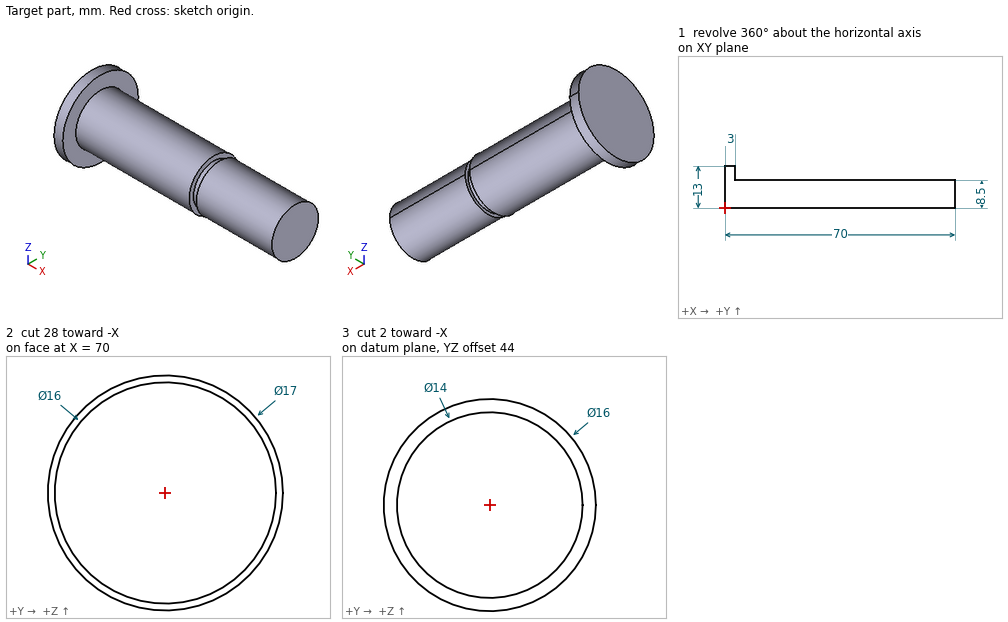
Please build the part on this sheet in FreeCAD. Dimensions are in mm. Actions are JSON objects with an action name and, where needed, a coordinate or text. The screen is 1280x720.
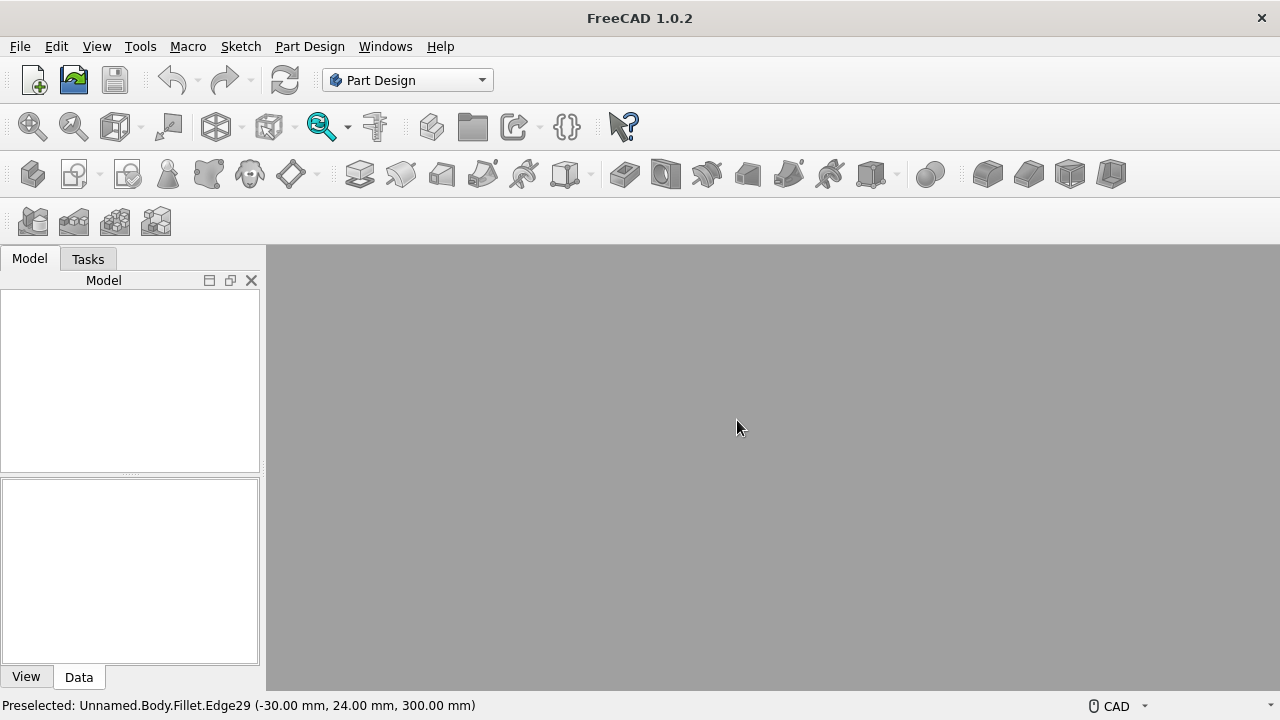
{"action": "key", "text": "ctrl+n"}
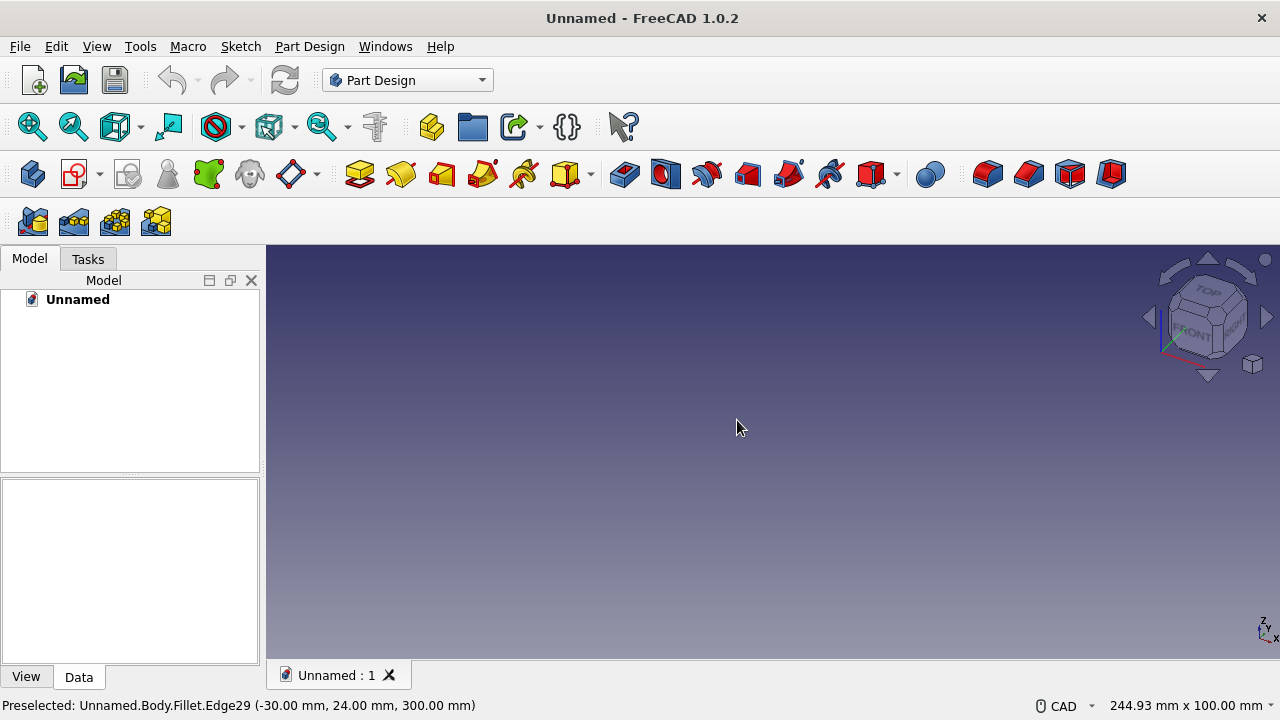
{"action": "left_click", "coordinate": [74, 174]}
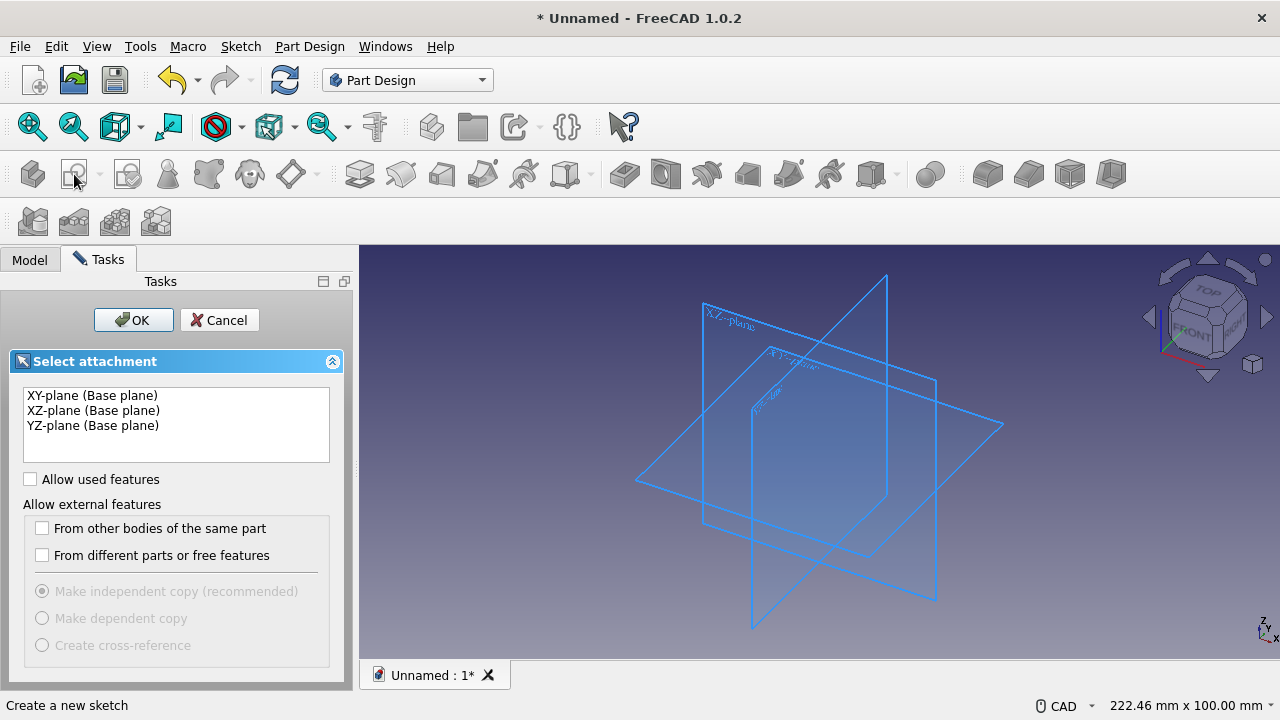
{"action": "left_click", "coordinate": [84, 396]}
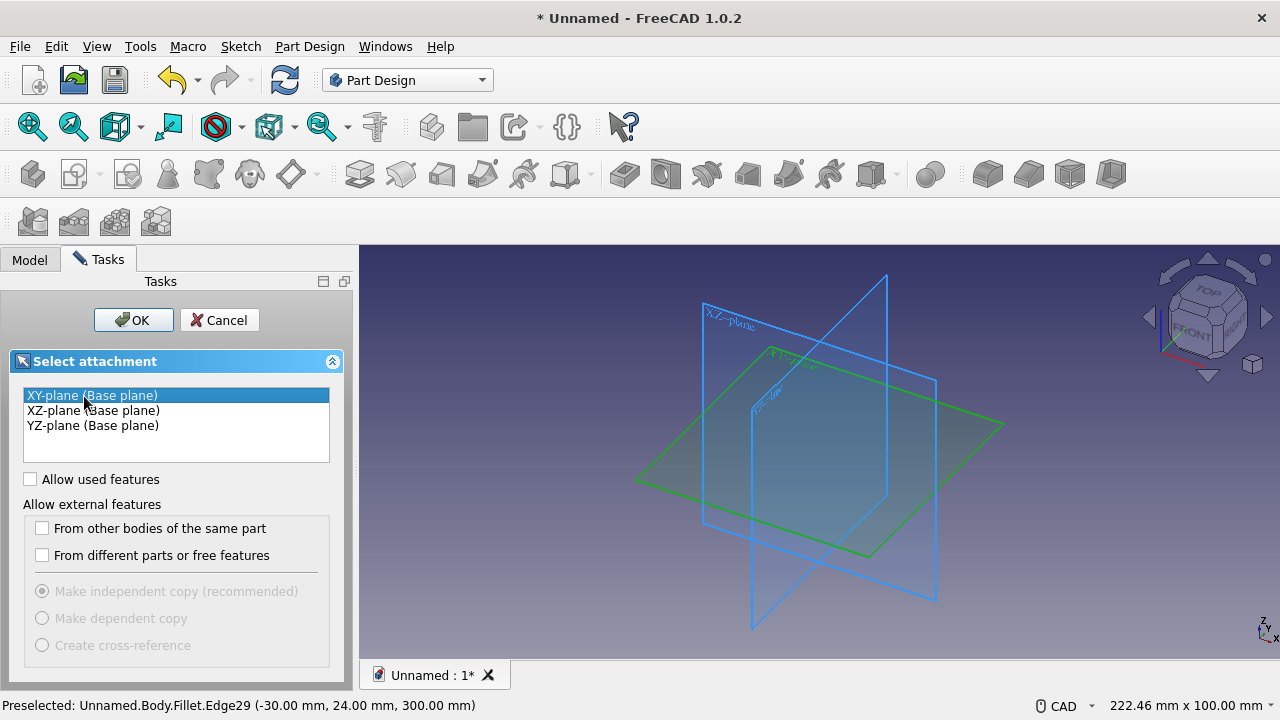
{"action": "left_click", "coordinate": [134, 320]}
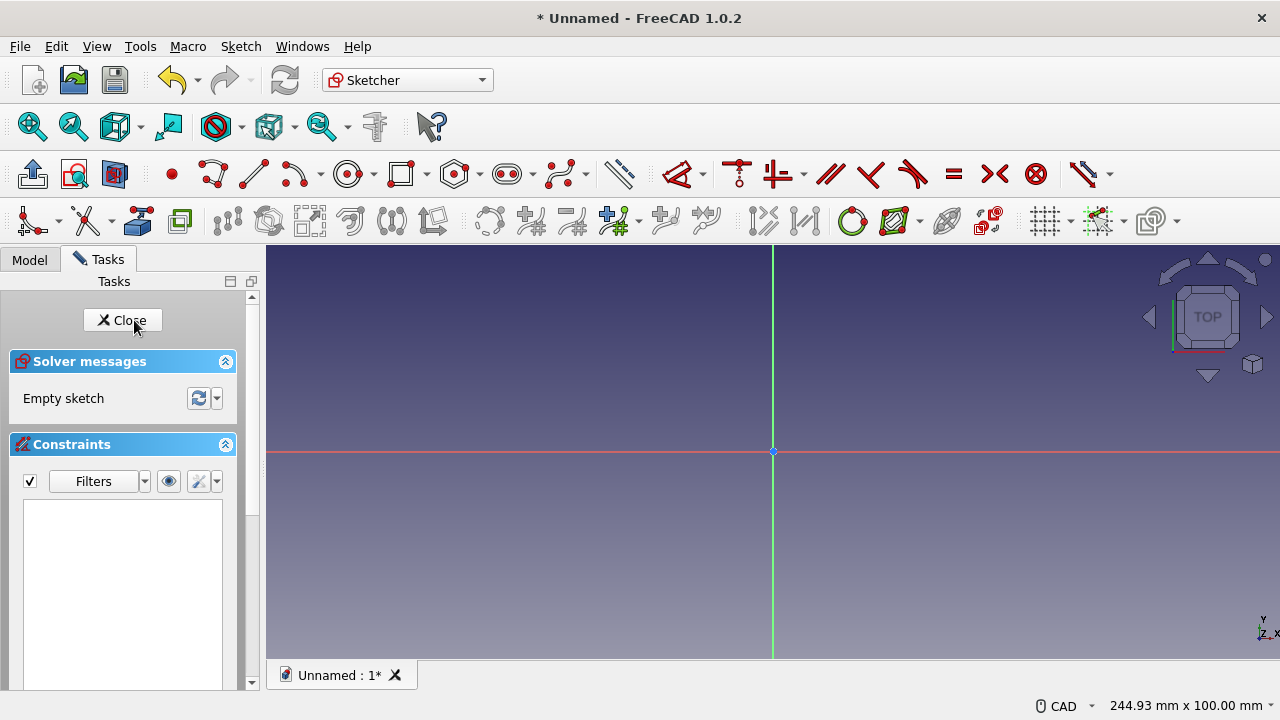
{"action": "scroll", "coordinate": [1115, 392], "scroll_direction": "up", "scroll_amount": 3}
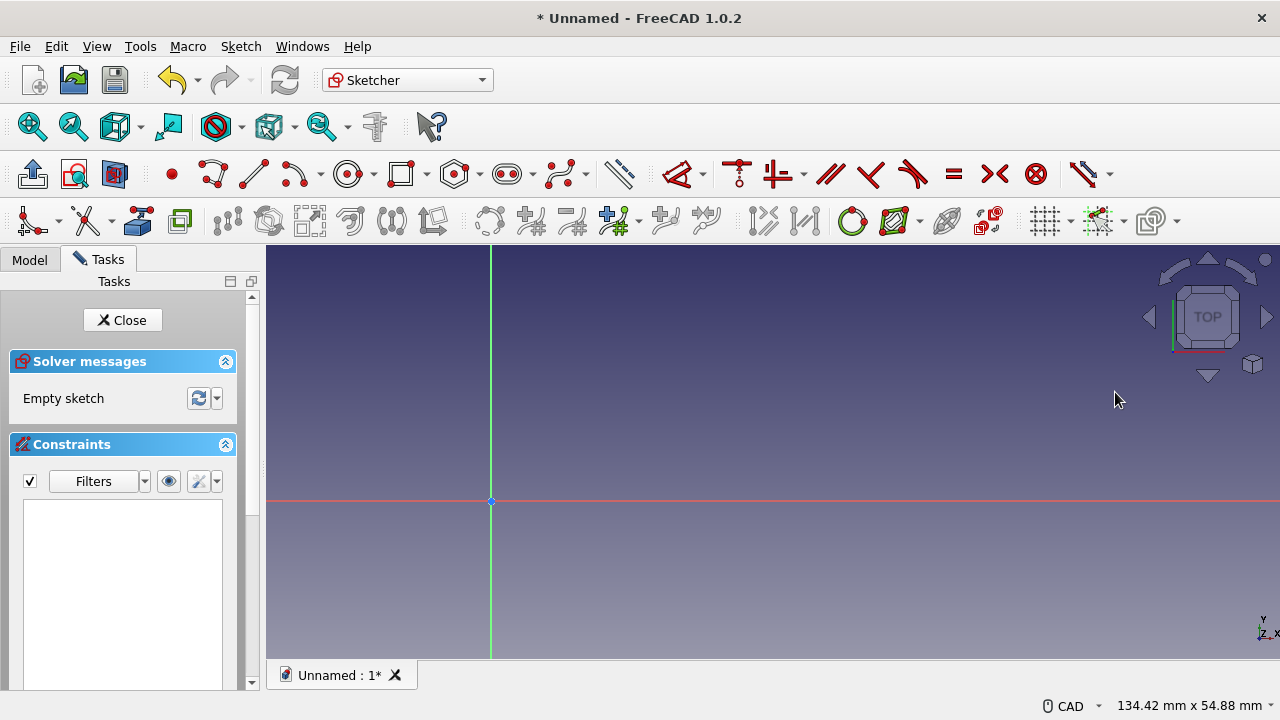
{"action": "key", "text": "g m"}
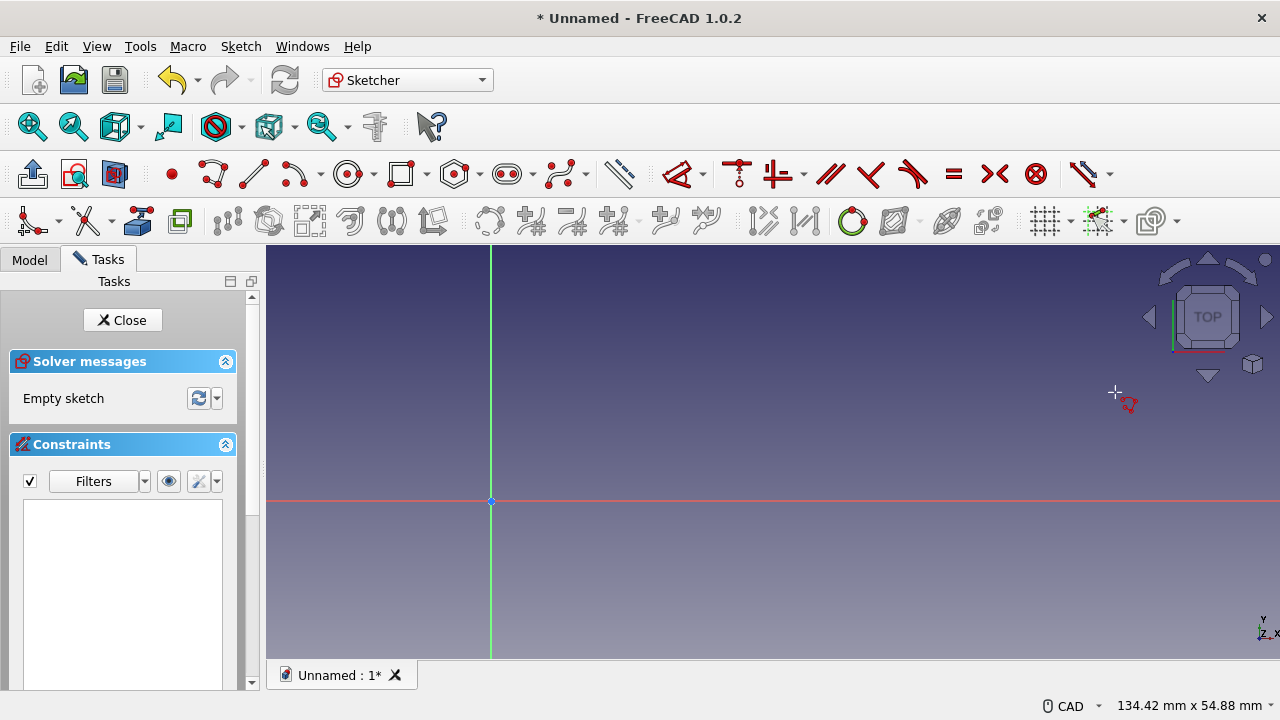
{"action": "left_click", "coordinate": [491, 501]}
{"action": "left_click", "coordinate": [1019, 492]}
{"action": "left_click", "coordinate": [1019, 437]}
{"action": "left_click", "coordinate": [514, 437]}
{"action": "left_click", "coordinate": [514, 403]}
{"action": "left_click", "coordinate": [500, 403]}
{"action": "left_click", "coordinate": [491, 501]}
{"action": "key", "text": "Escape"}
{"action": "key", "text": "Escape"}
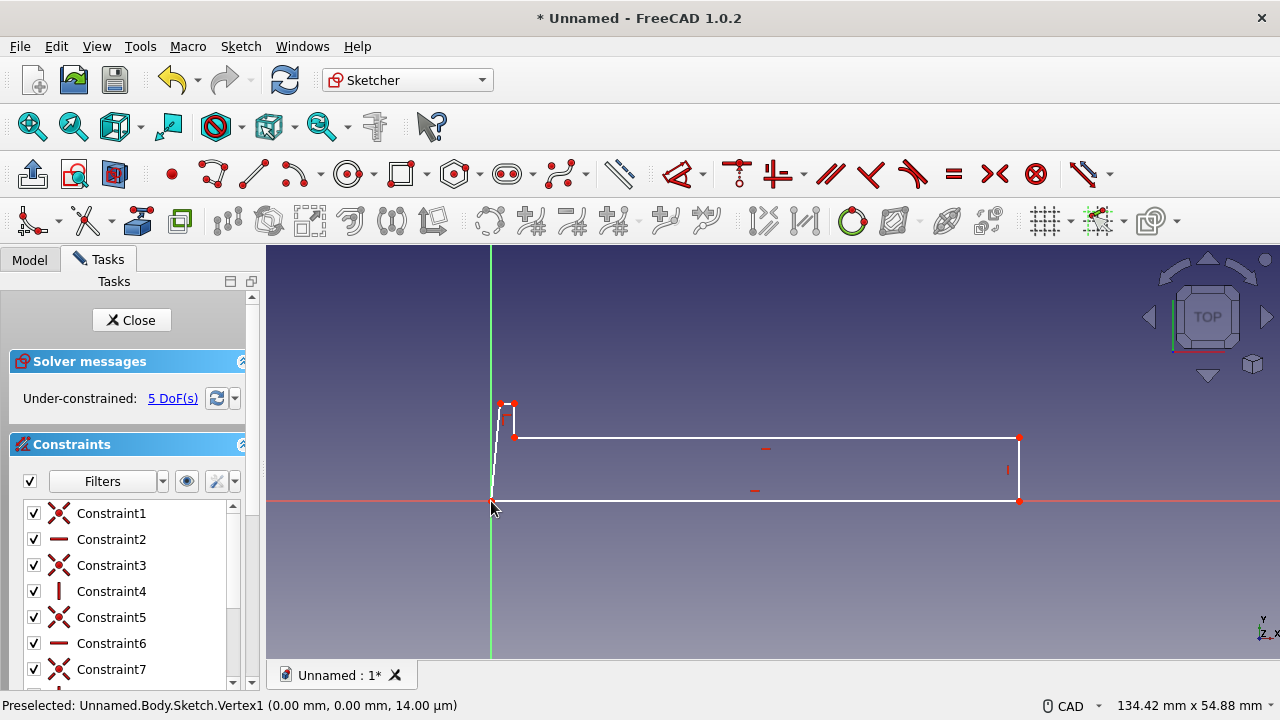
{"action": "left_click", "coordinate": [494, 472]}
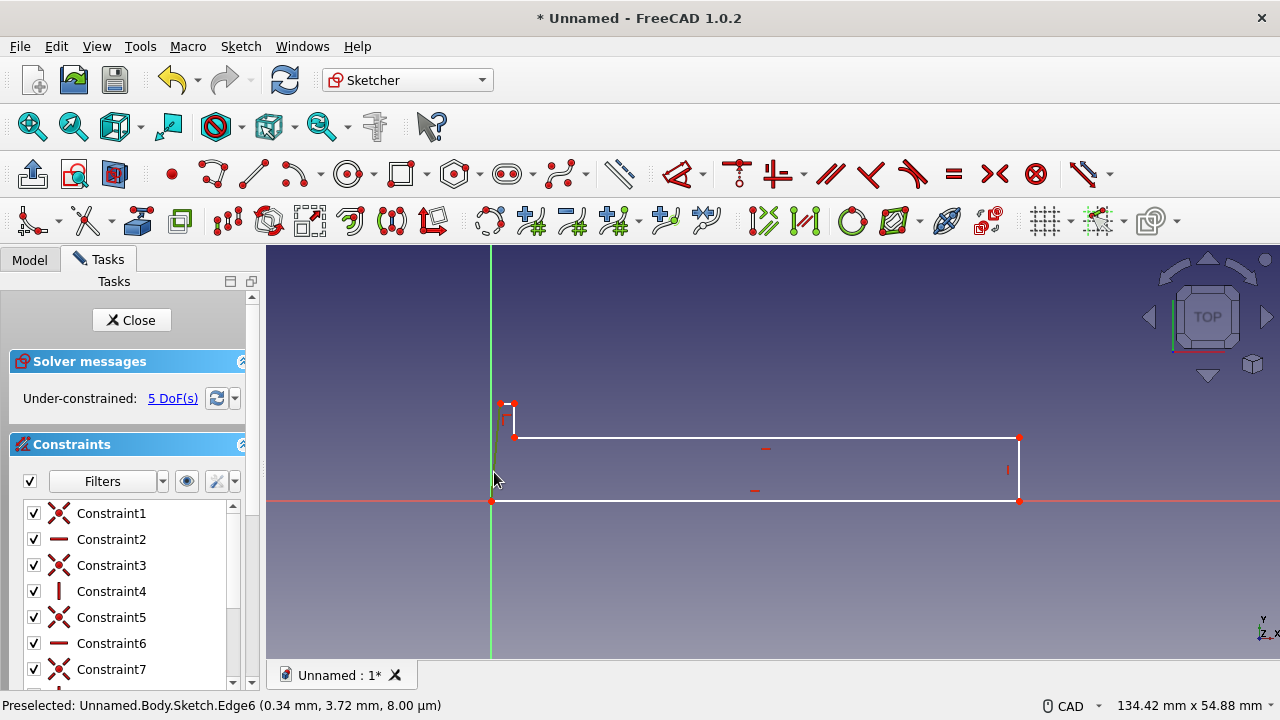
{"action": "key", "text": "v"}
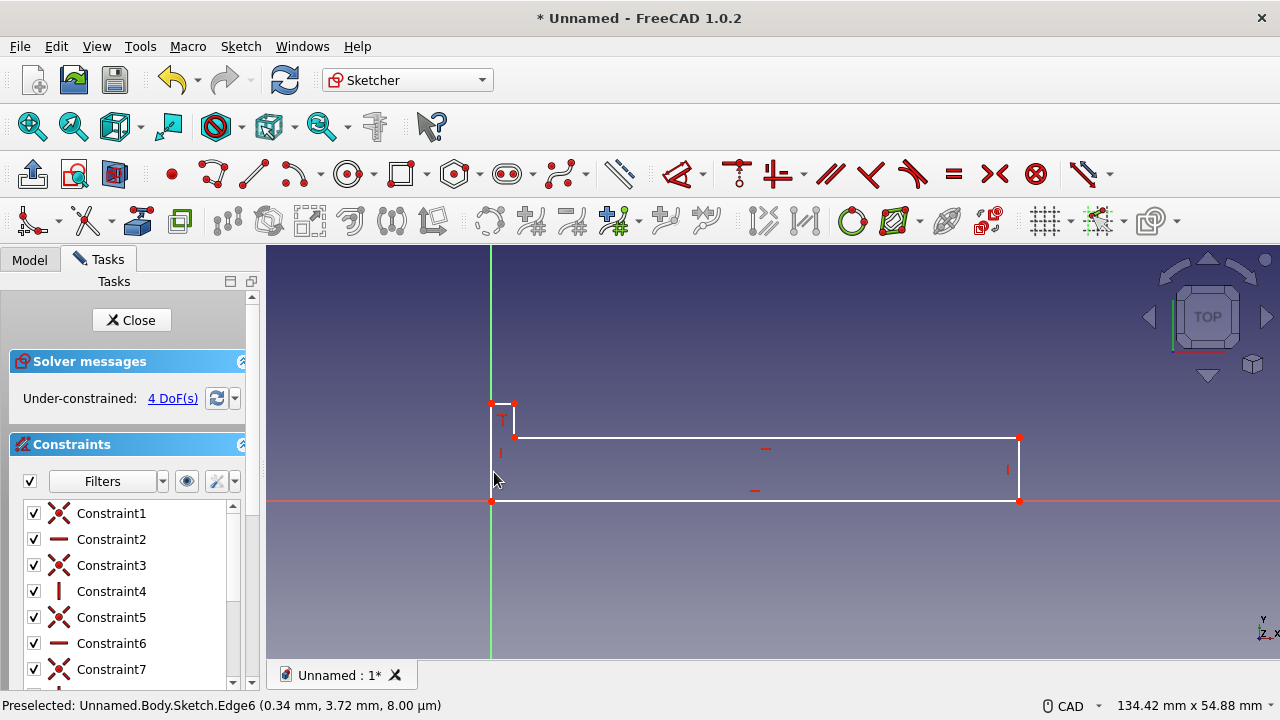
{"action": "scroll", "coordinate": [505, 404], "scroll_direction": "up", "scroll_amount": 3}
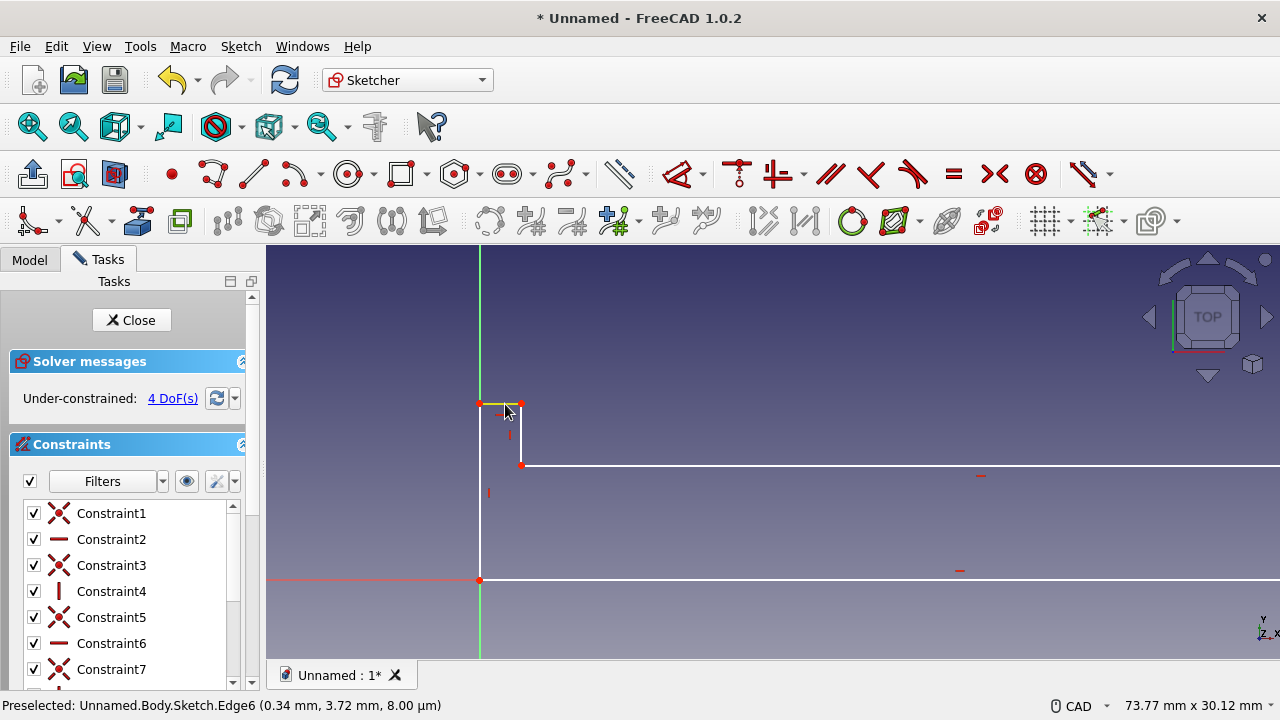
{"action": "left_click", "coordinate": [505, 404]}